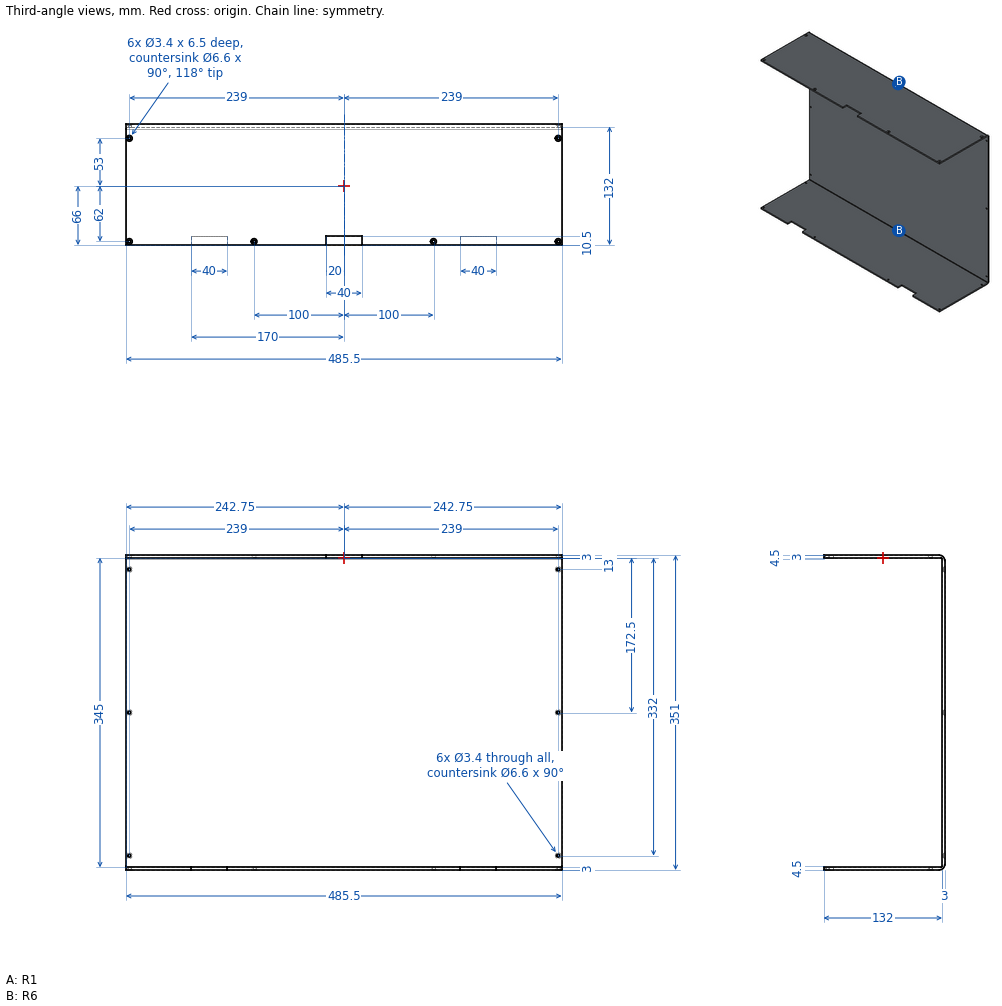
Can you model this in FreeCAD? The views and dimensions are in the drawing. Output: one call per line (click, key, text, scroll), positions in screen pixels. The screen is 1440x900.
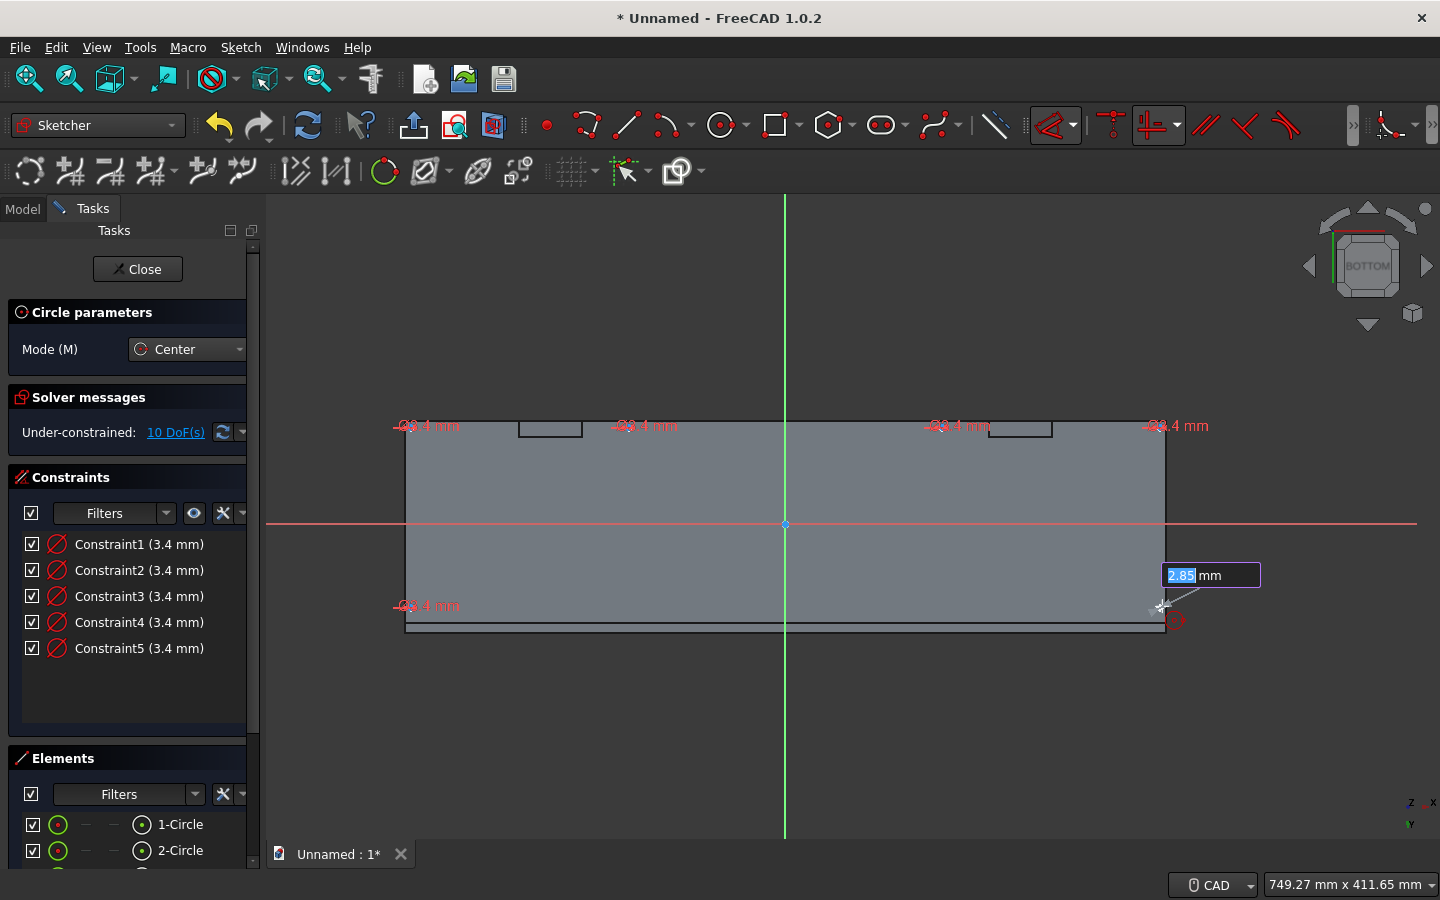
text(3.4)
key(Return)
key(Escape)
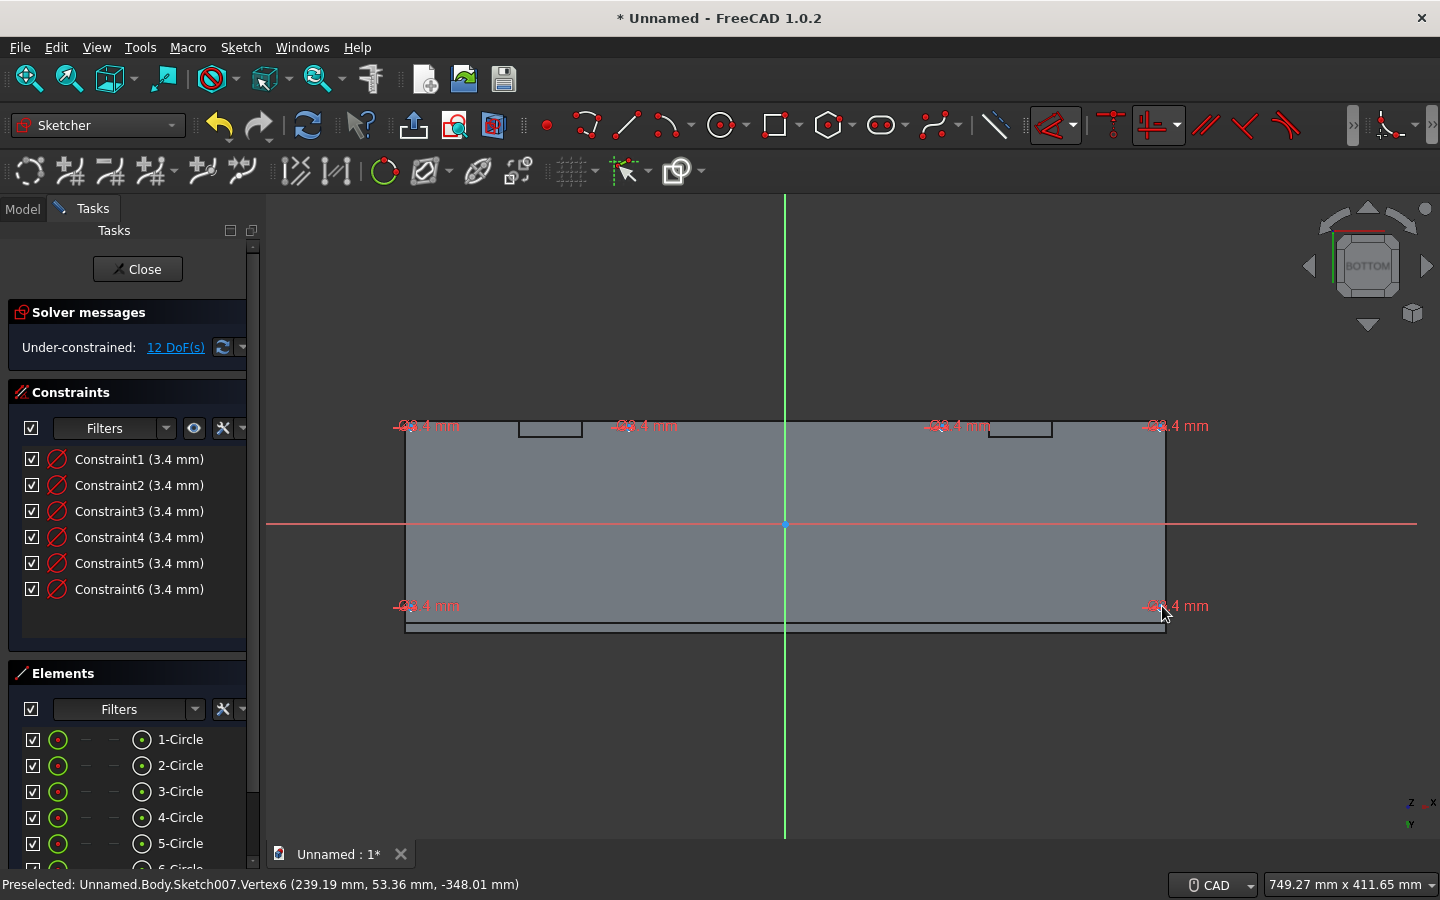
click(411, 608)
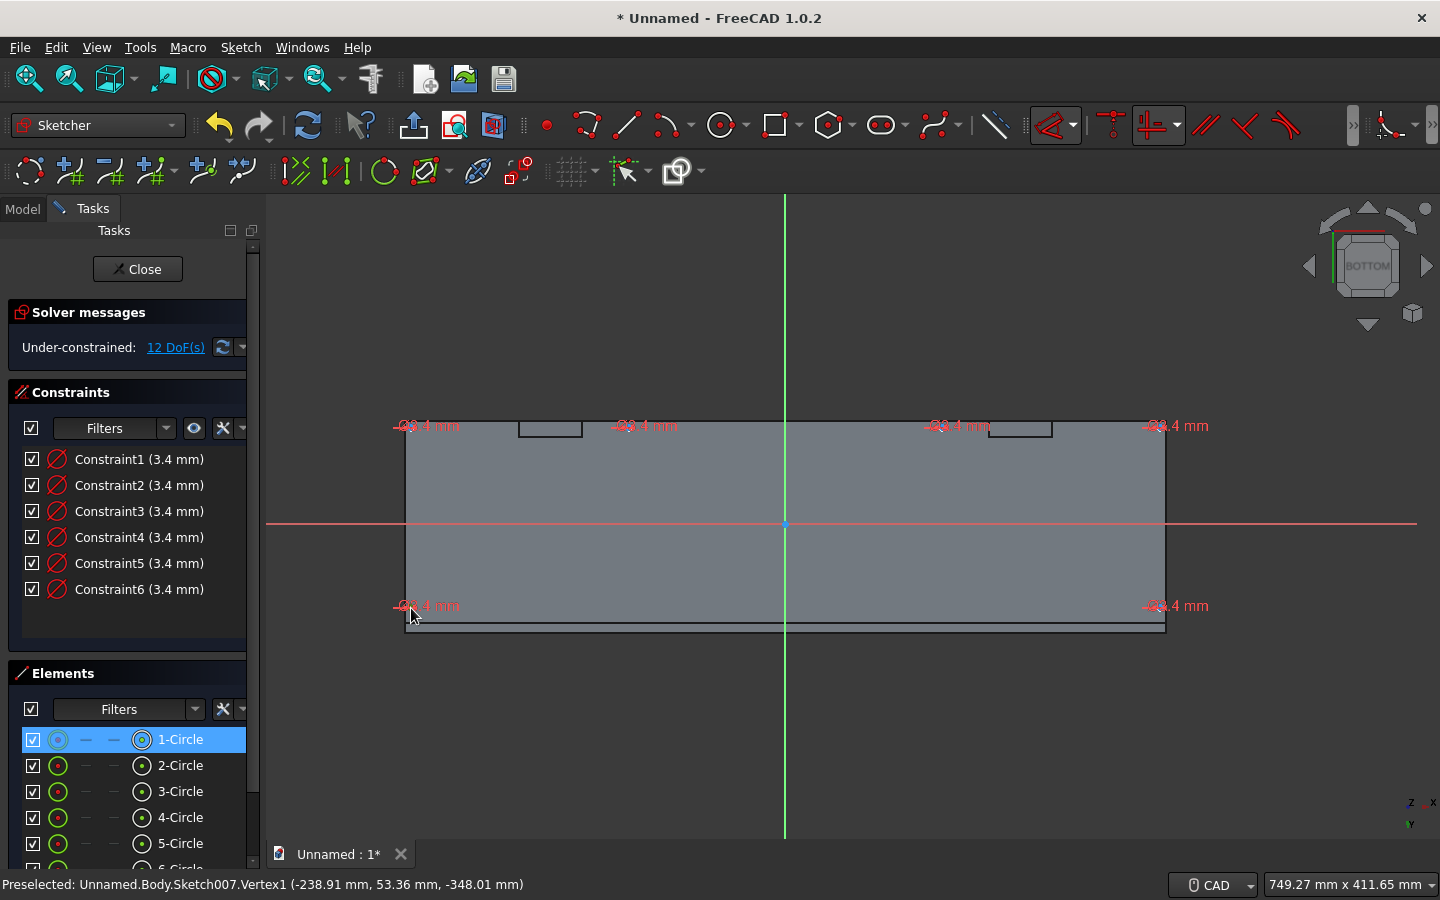
click(411, 428)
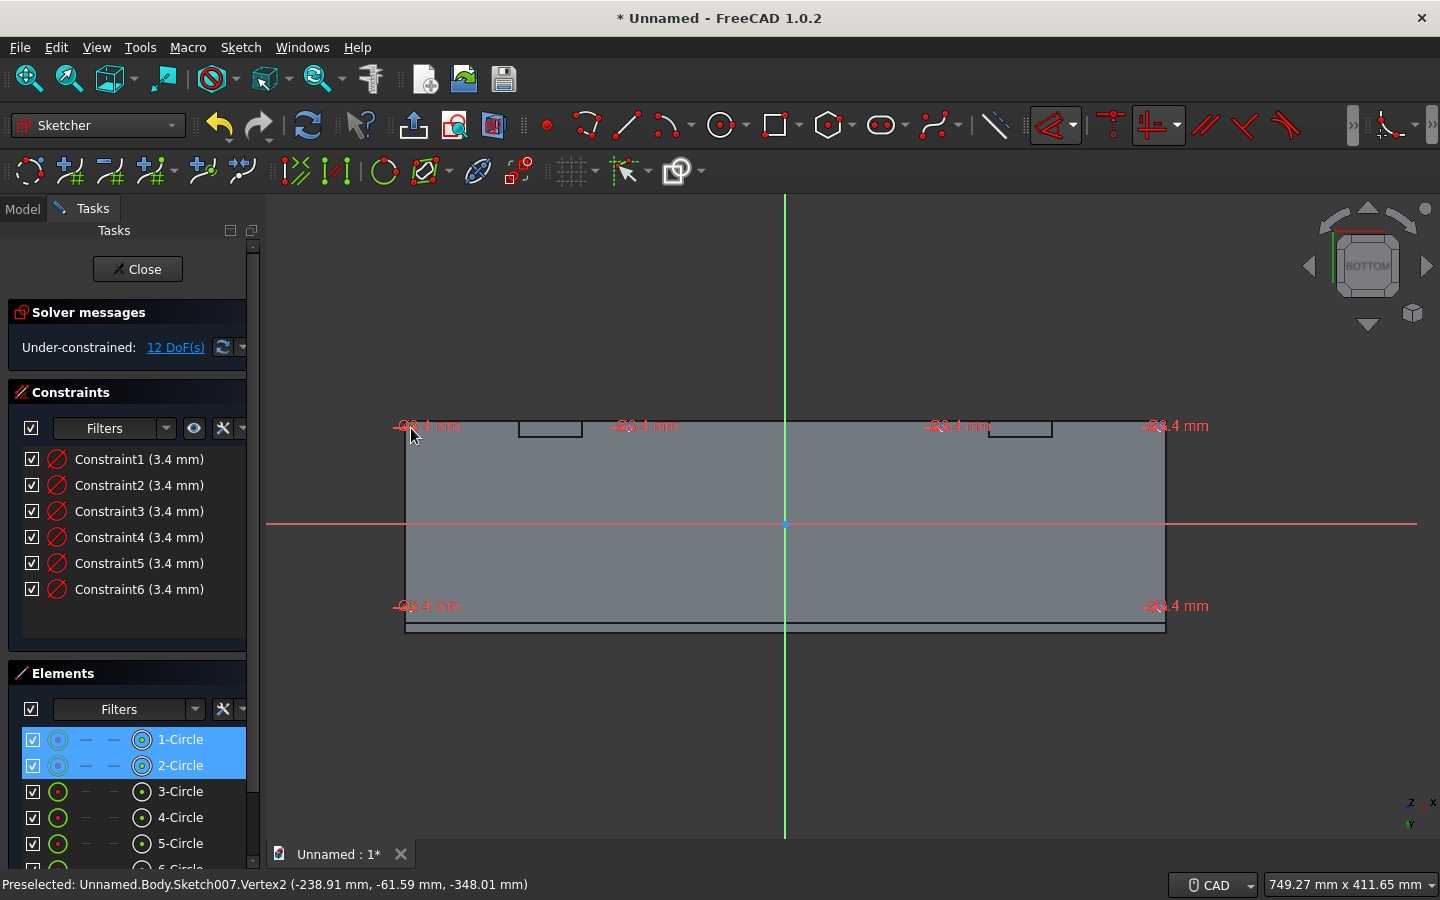
click(1180, 126)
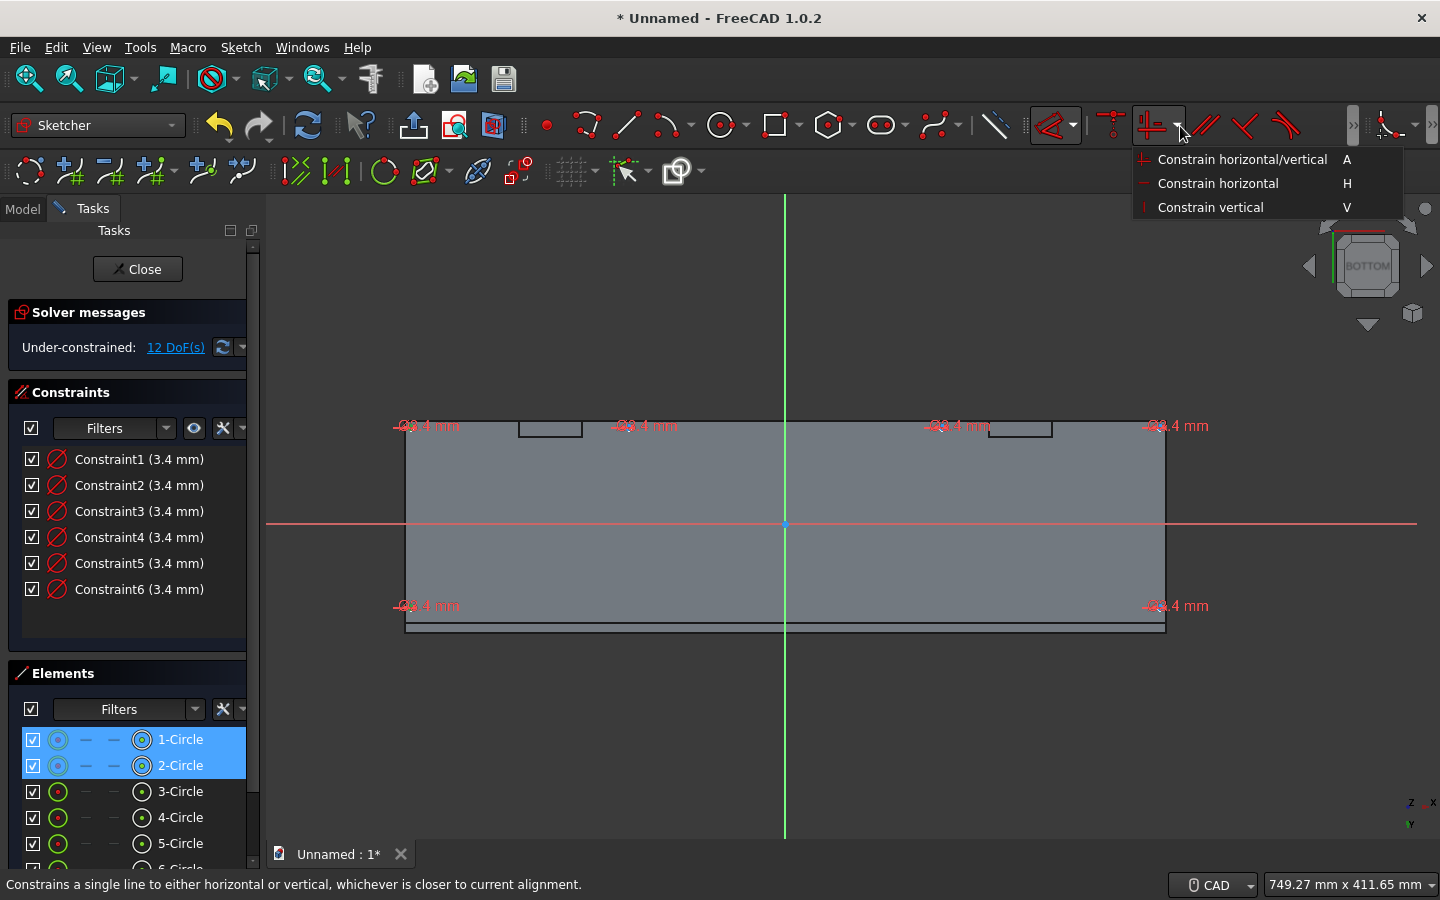
click(1268, 207)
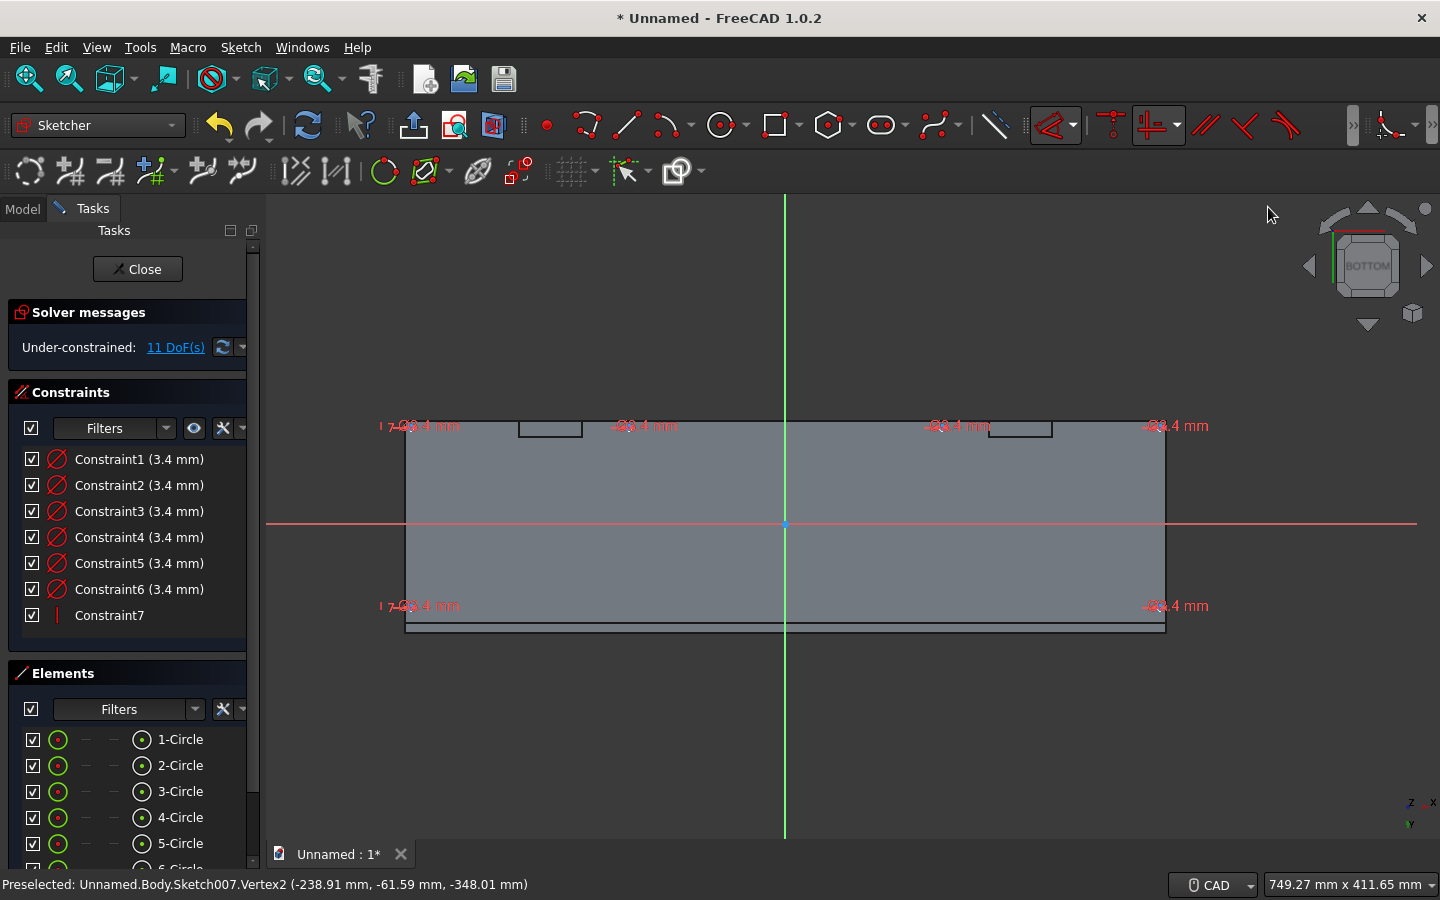
click(411, 428)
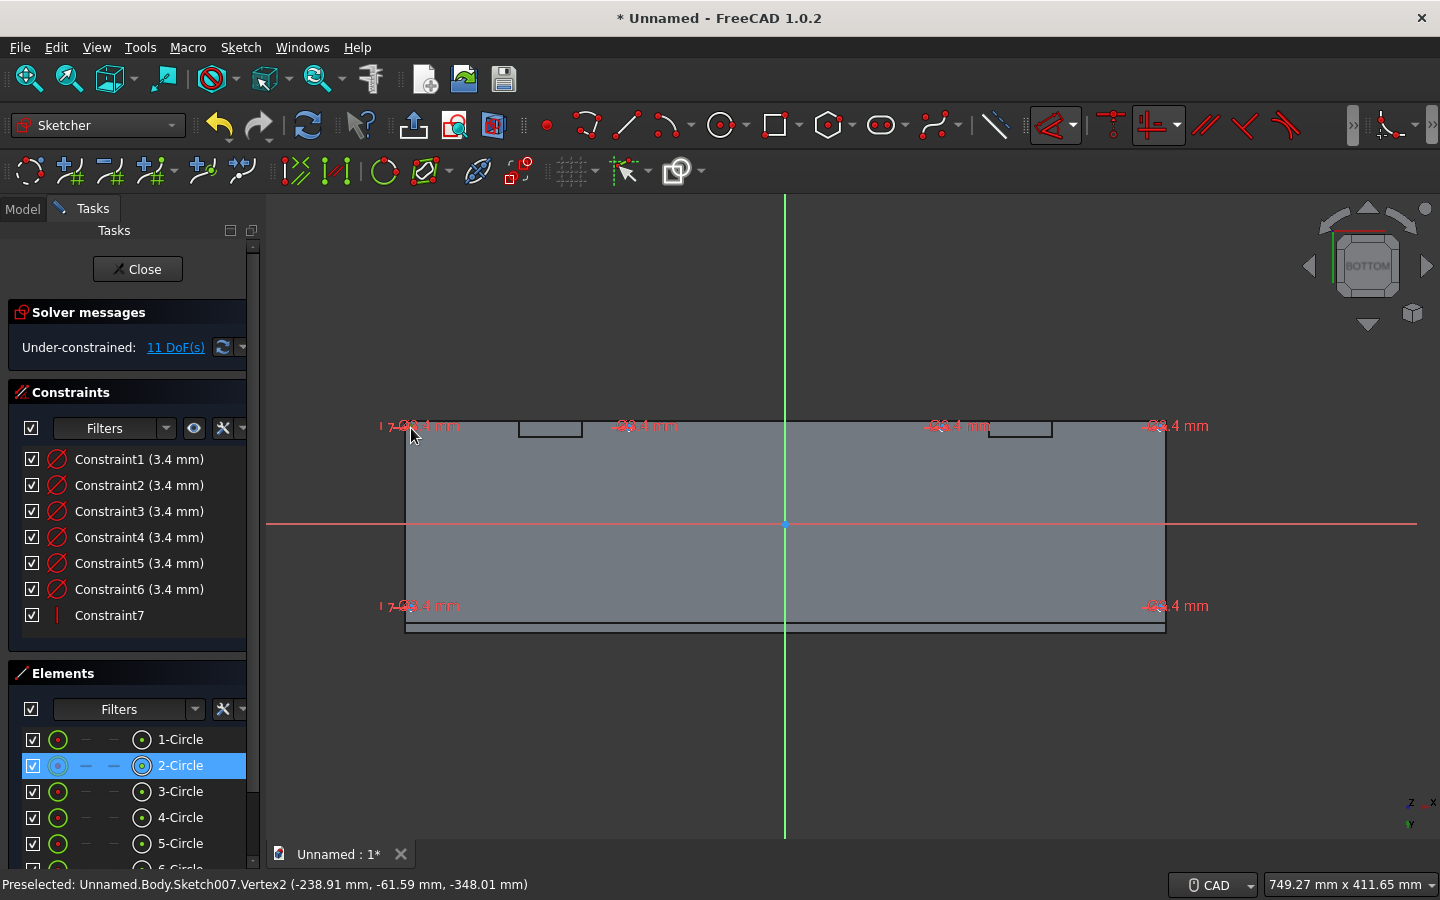
click(629, 428)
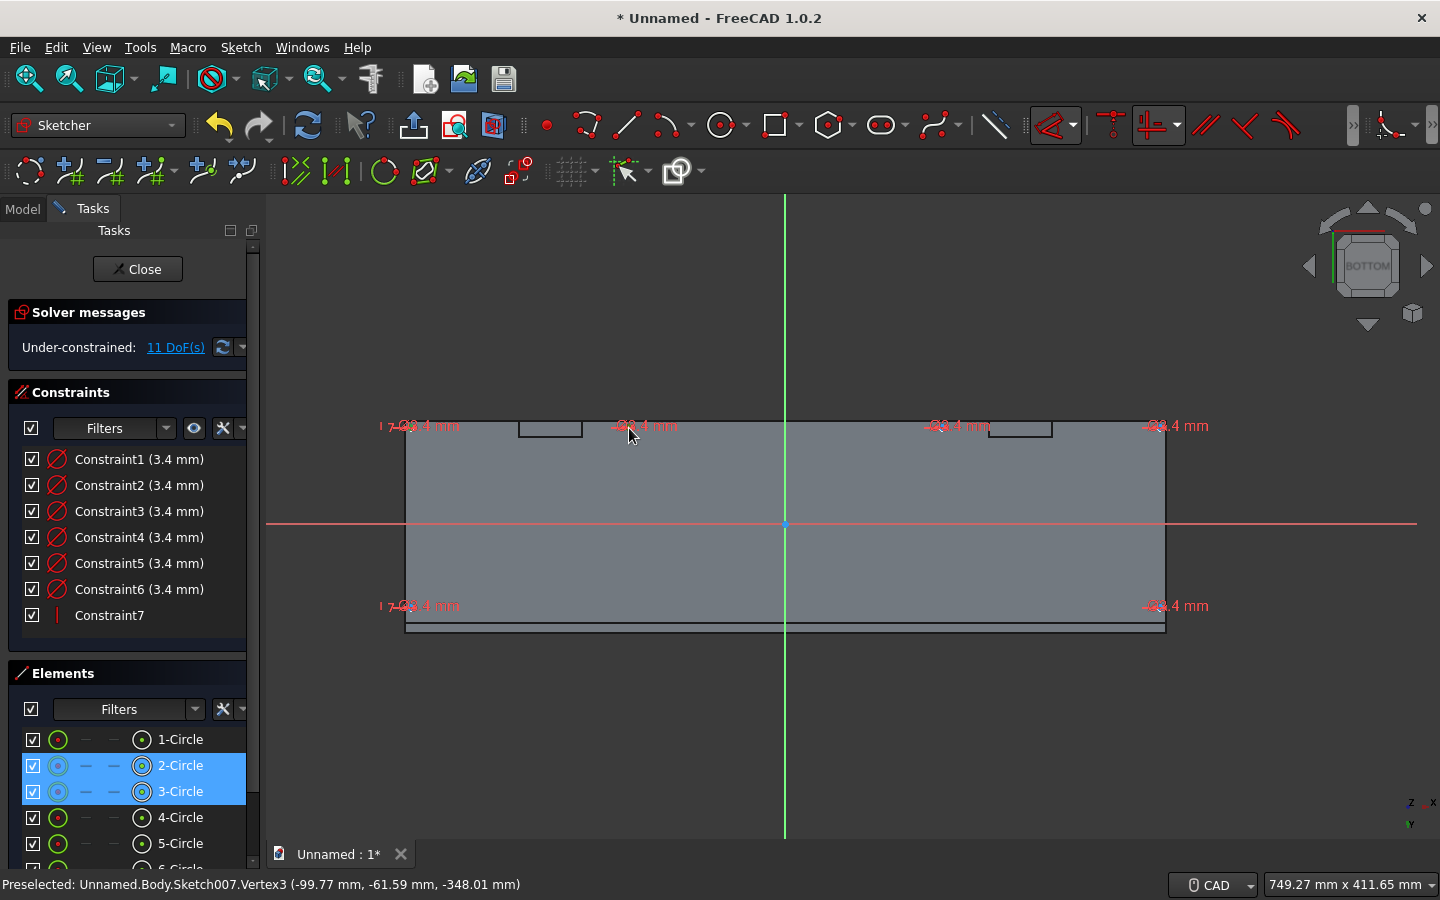
click(1180, 126)